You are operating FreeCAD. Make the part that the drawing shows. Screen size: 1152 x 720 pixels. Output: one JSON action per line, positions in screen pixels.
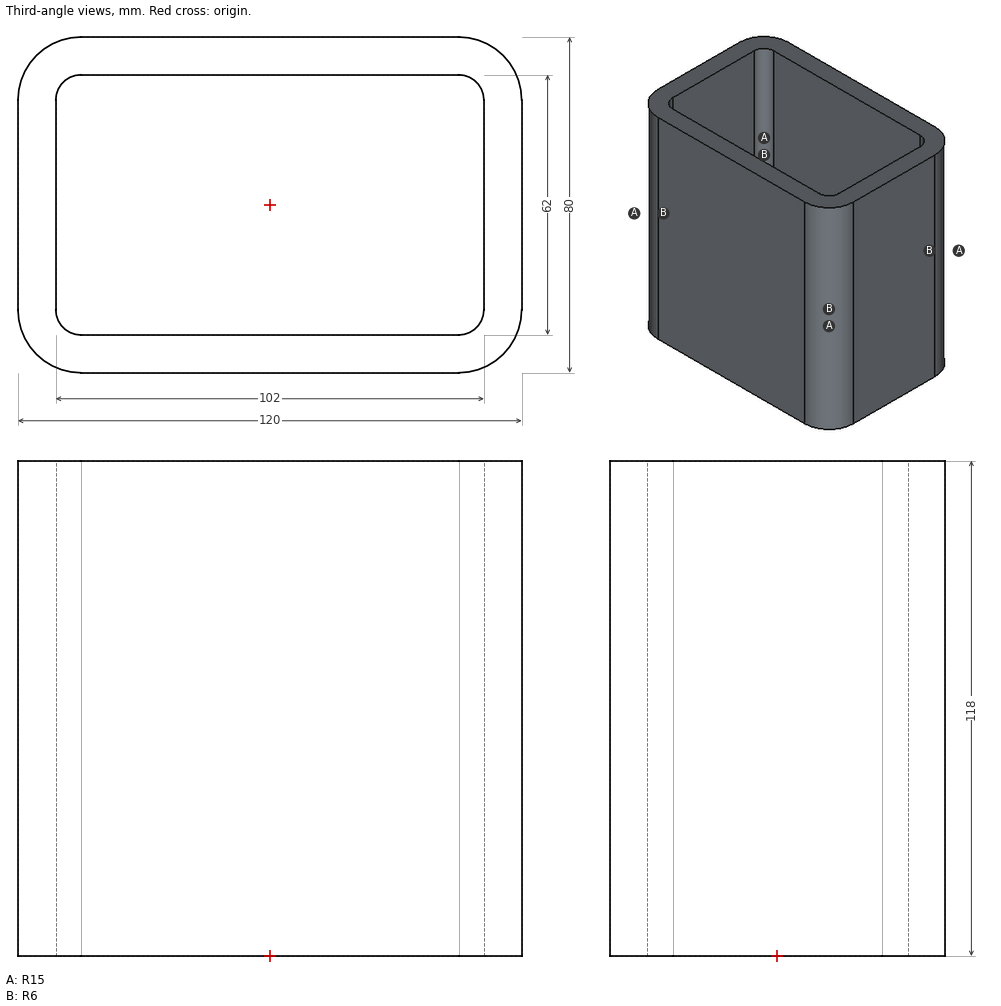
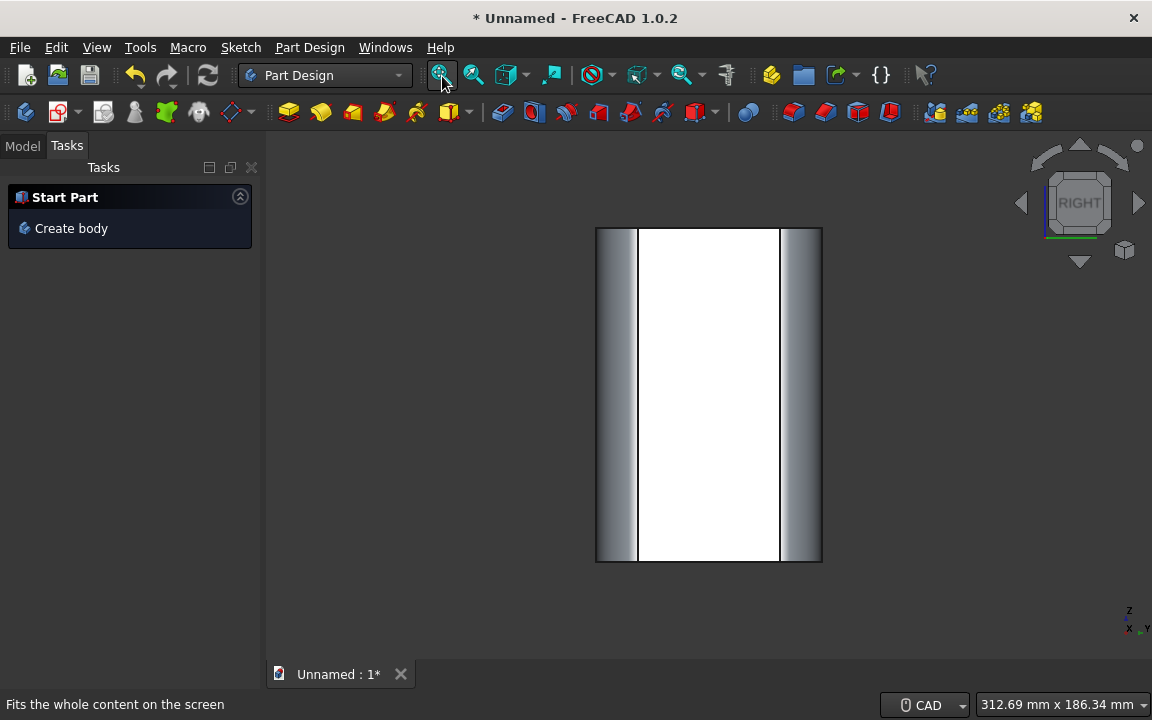
{"action": "key", "text": "5"}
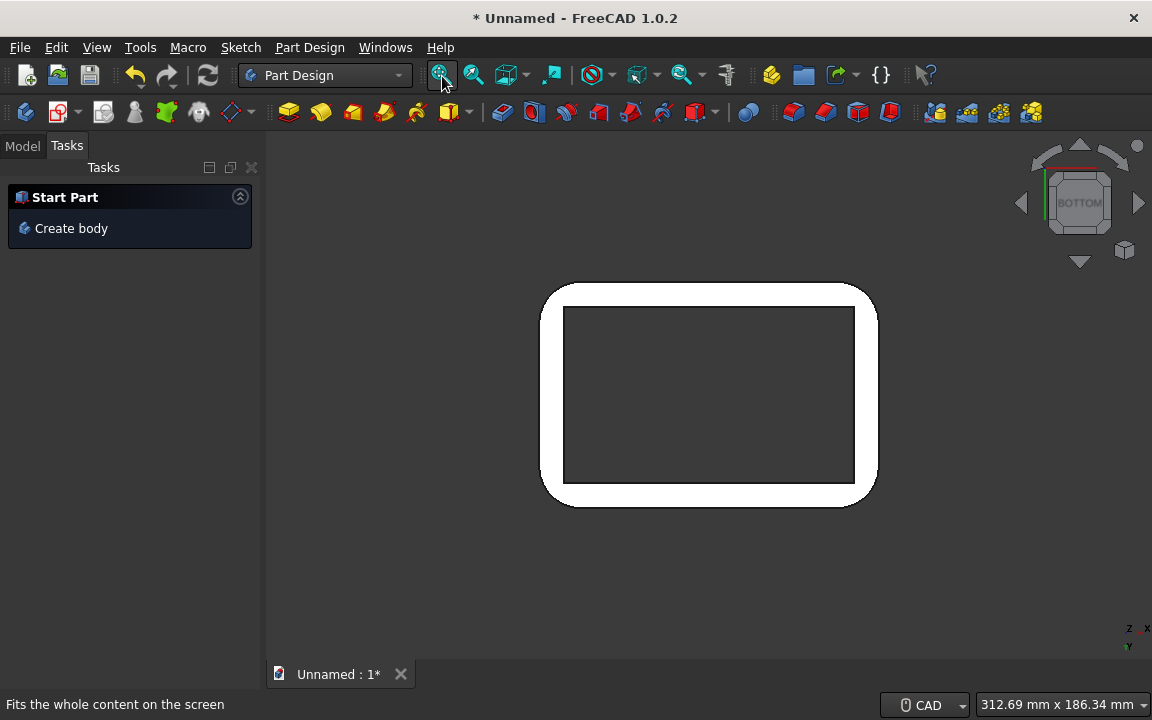
{"action": "left_click", "coordinate": [442, 76]}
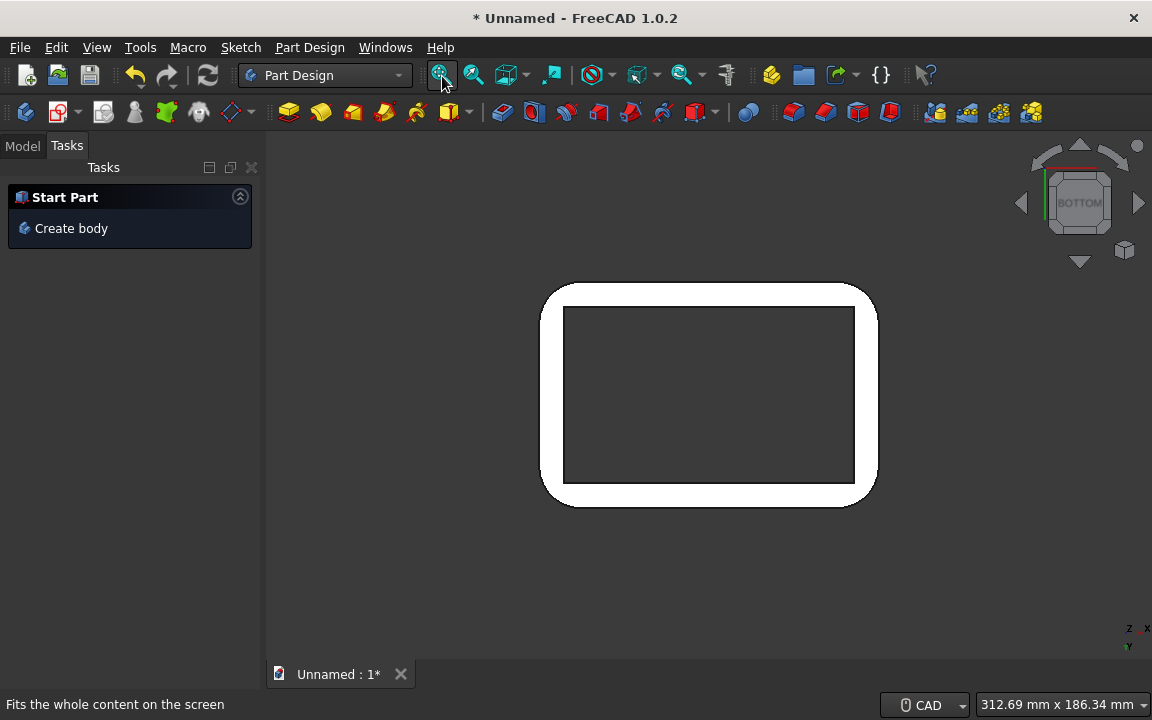
{"action": "key", "text": "4"}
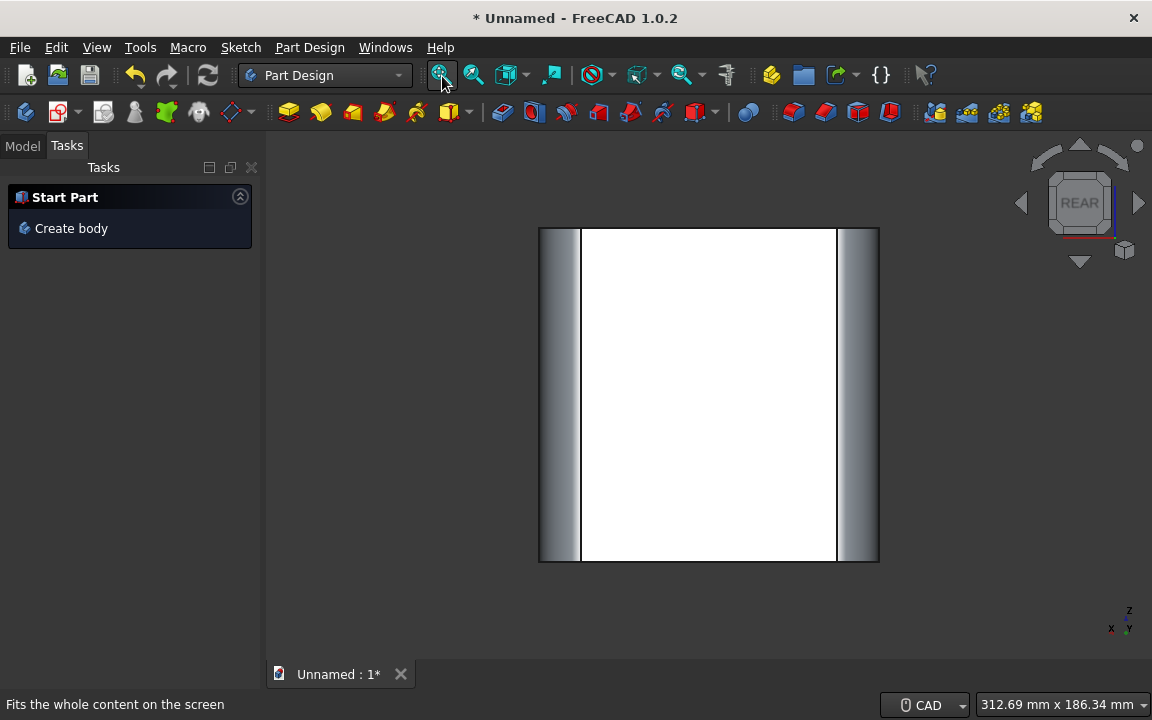
{"action": "key", "text": "6"}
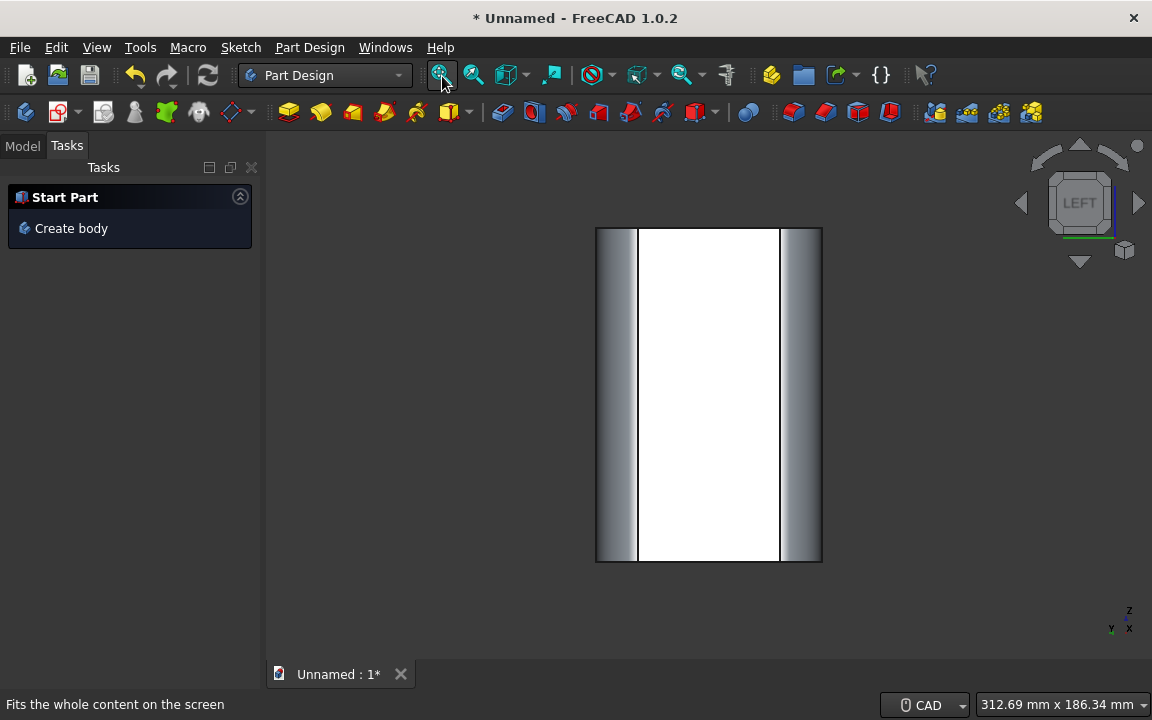
{"action": "key", "text": "v 3"}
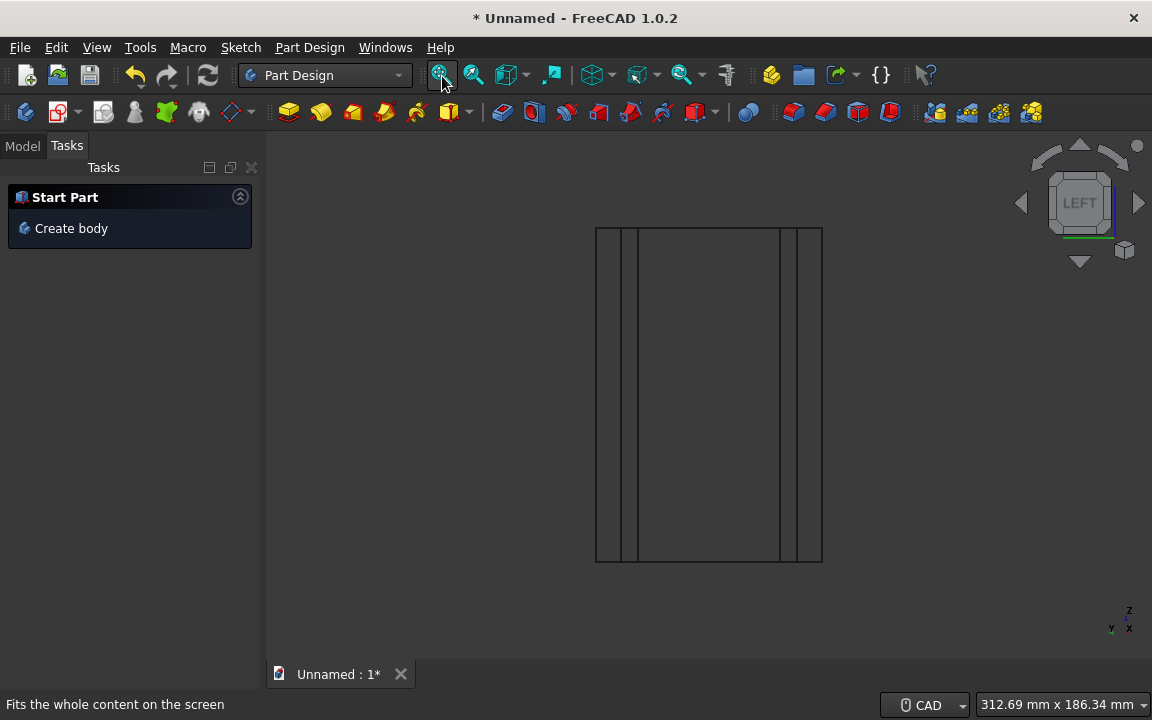
{"action": "key", "text": "0"}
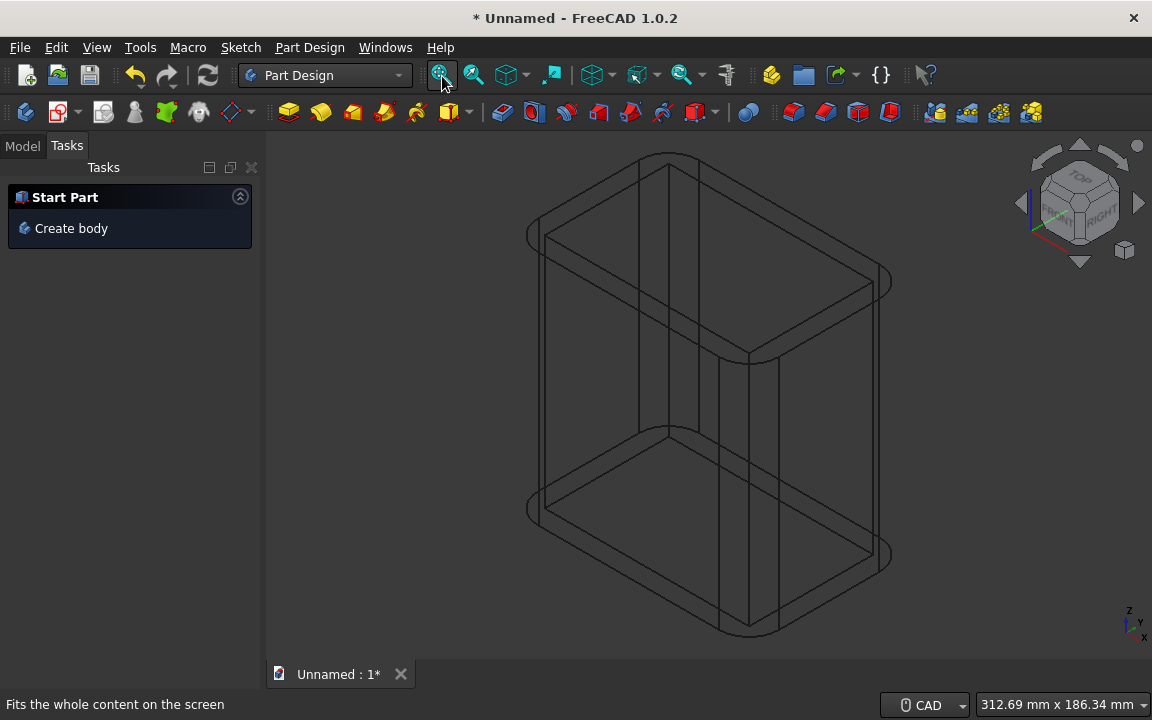
{"action": "left_click", "coordinate": [669, 272]}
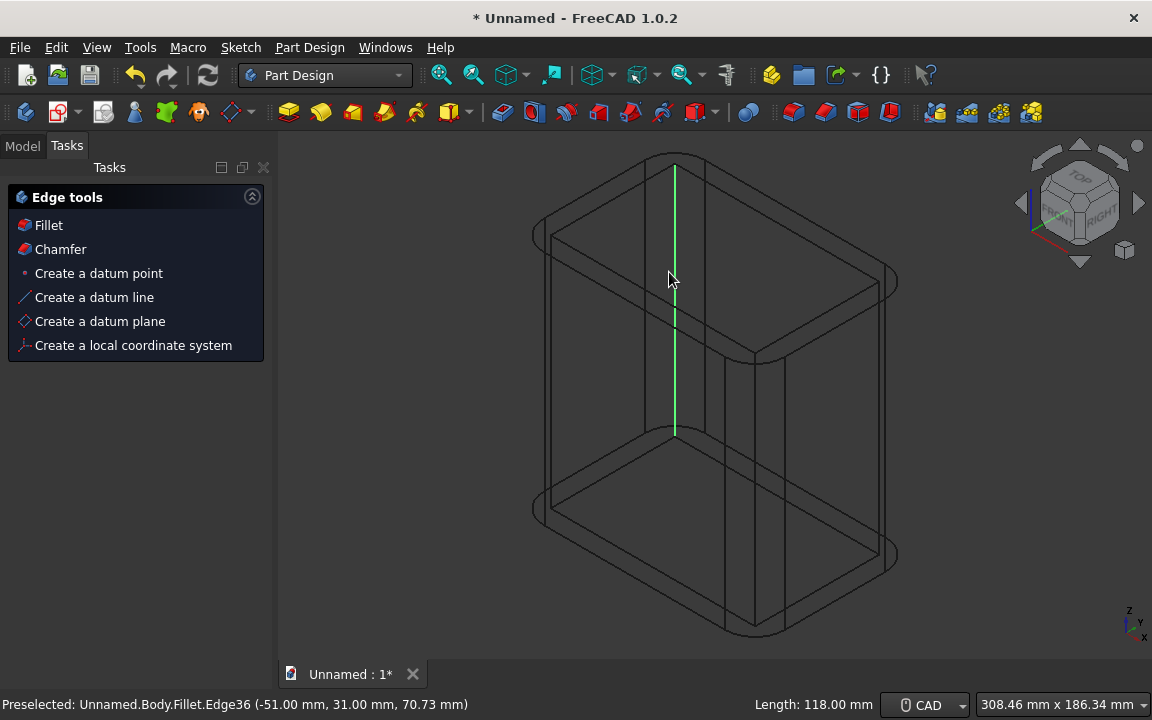
{"action": "left_click", "coordinate": [551, 371], "text": "ctrl"}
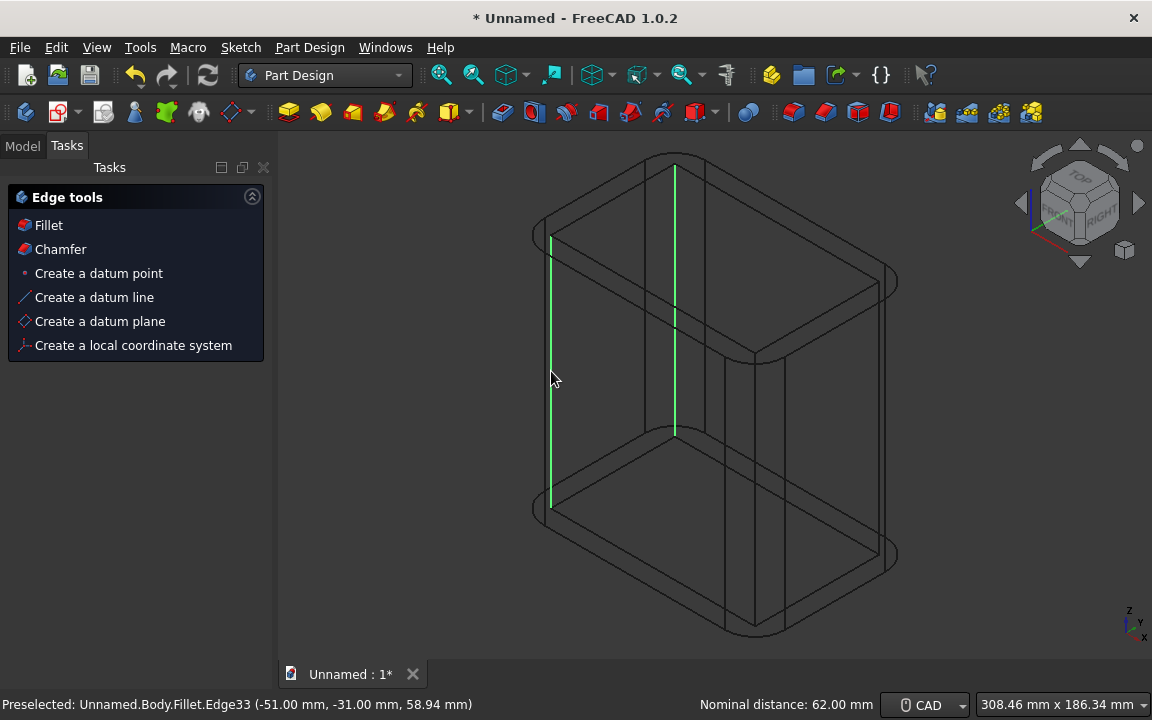
{"action": "left_click", "coordinate": [755, 489], "text": "ctrl"}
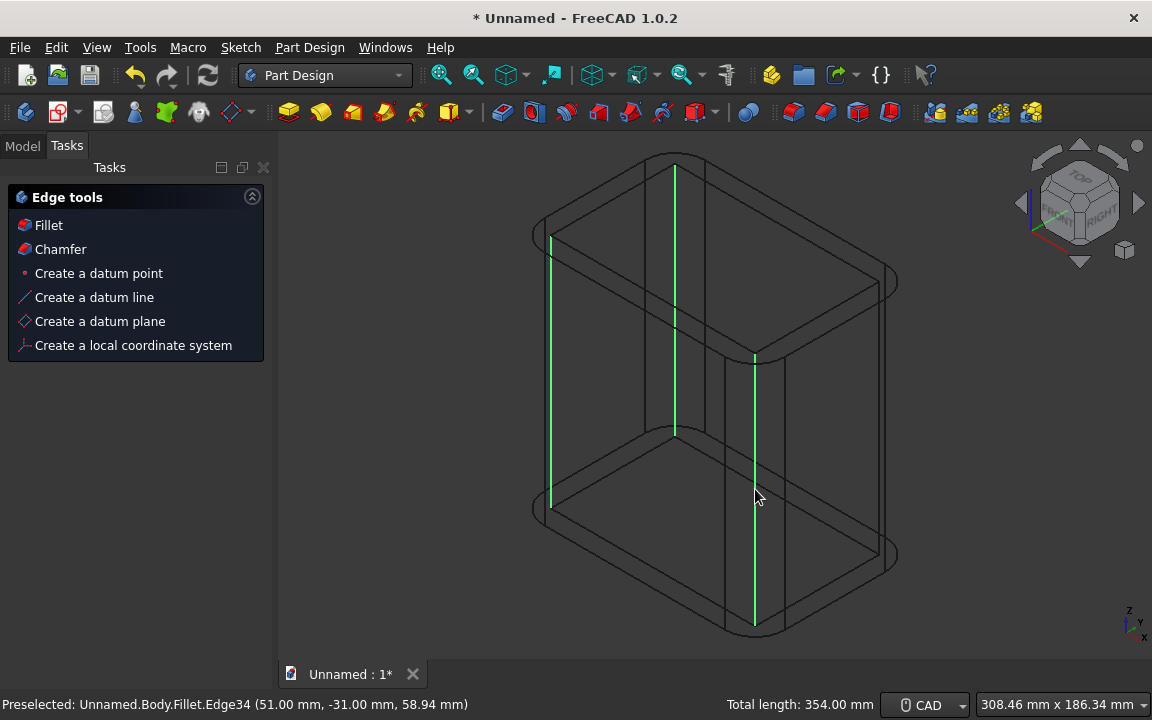
{"action": "left_click", "coordinate": [879, 417], "text": "ctrl"}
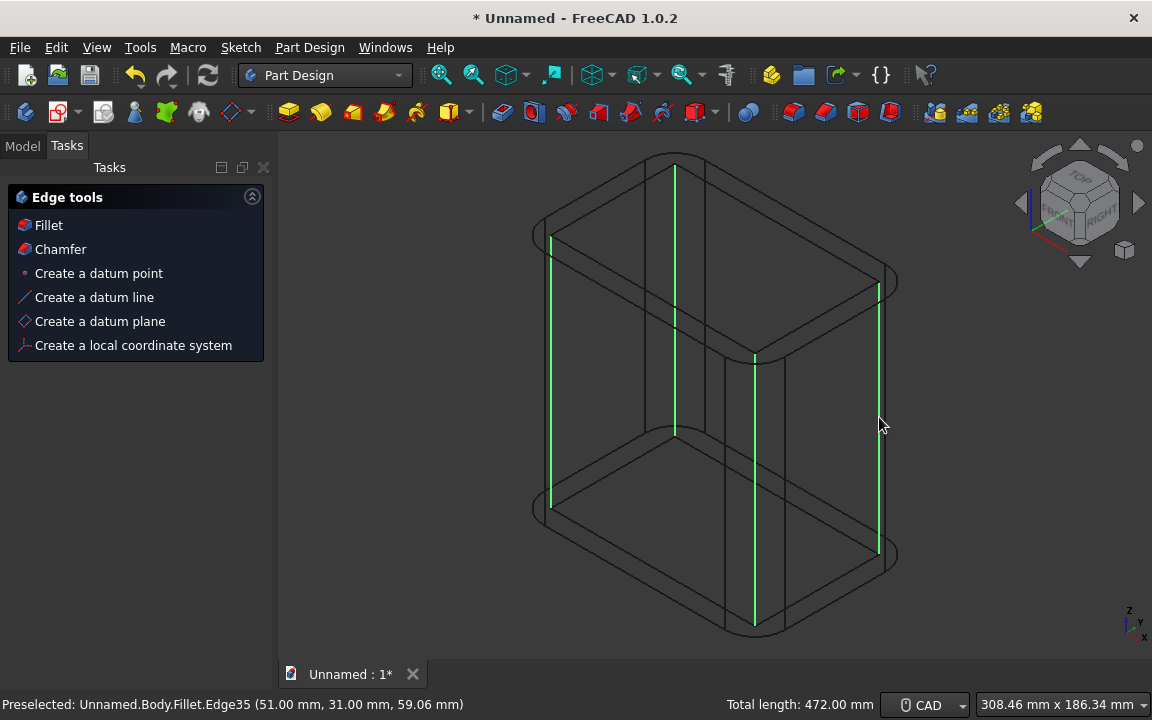
{"action": "key", "text": "v 1"}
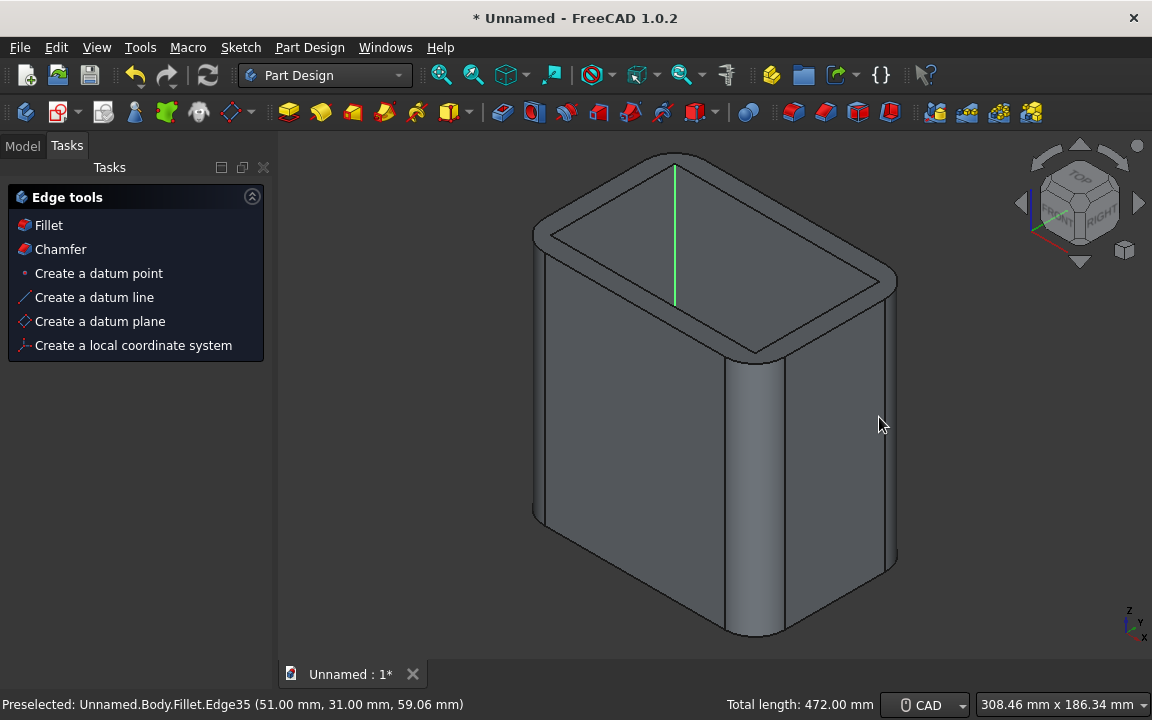
{"action": "left_click", "coordinate": [794, 112]}